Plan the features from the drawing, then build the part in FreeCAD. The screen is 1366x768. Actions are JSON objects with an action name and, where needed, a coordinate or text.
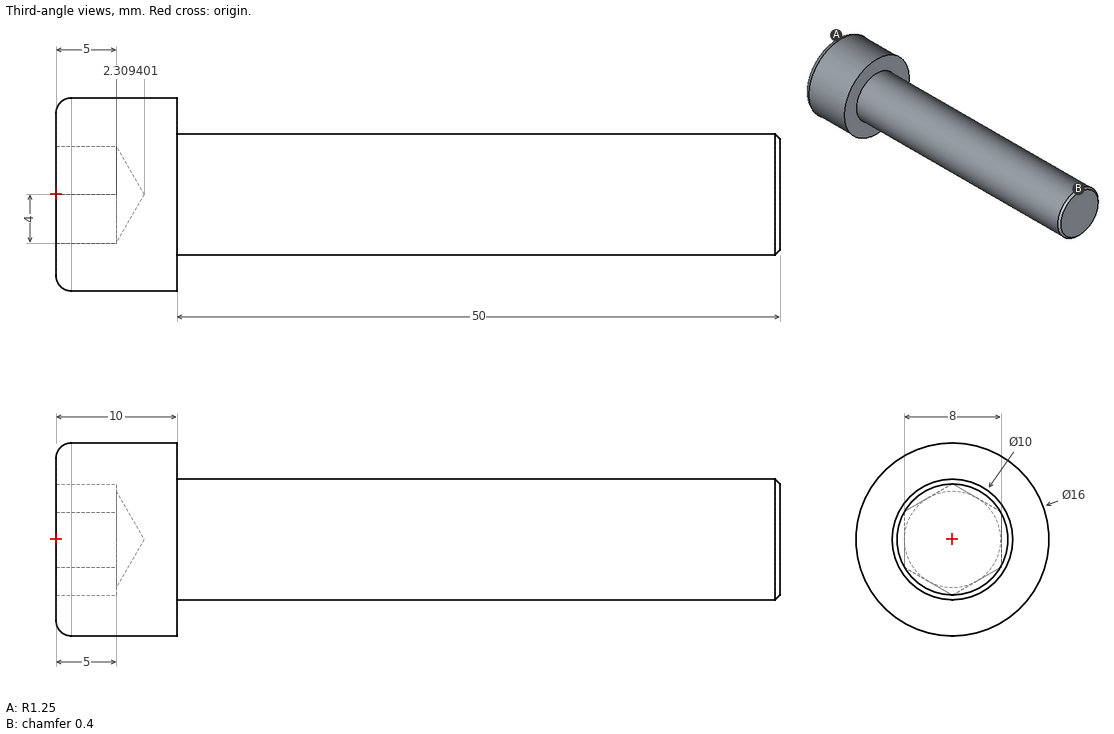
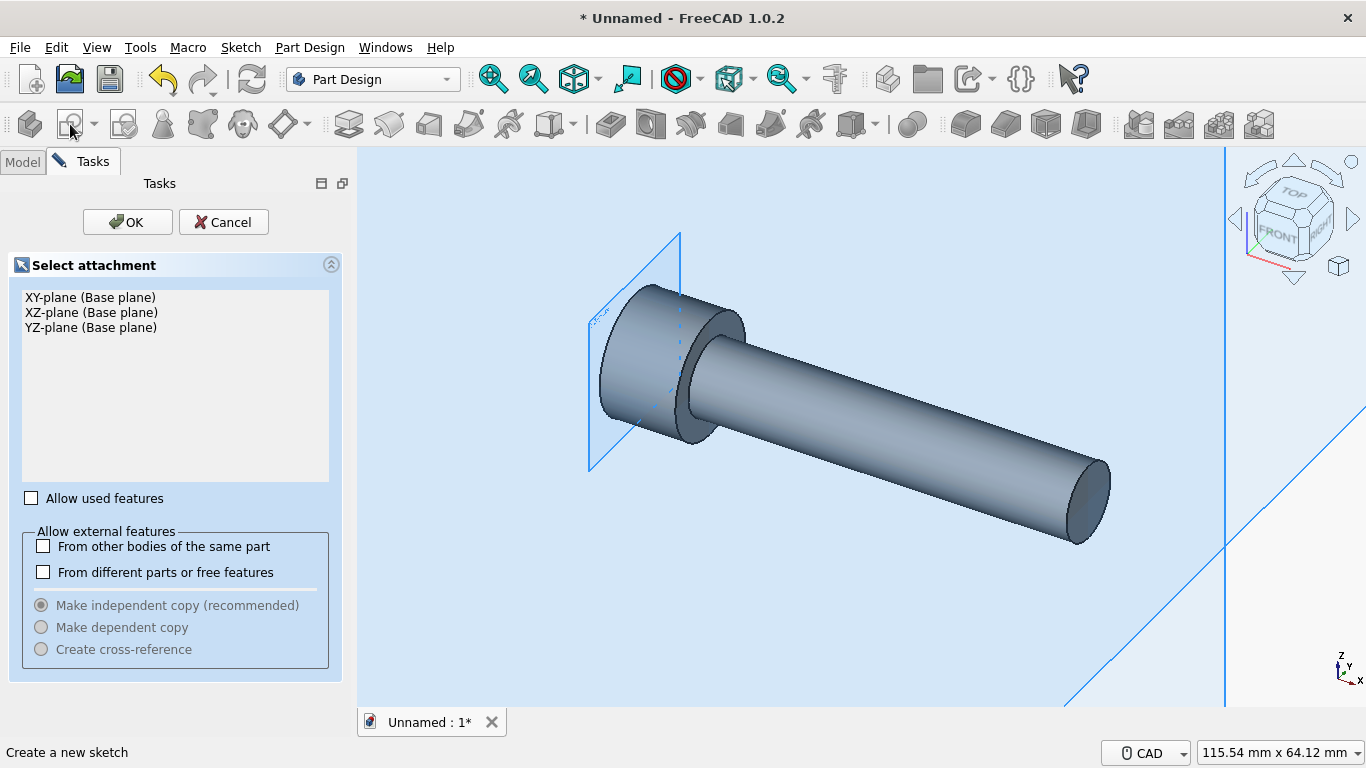
{"action": "left_click", "coordinate": [82, 328]}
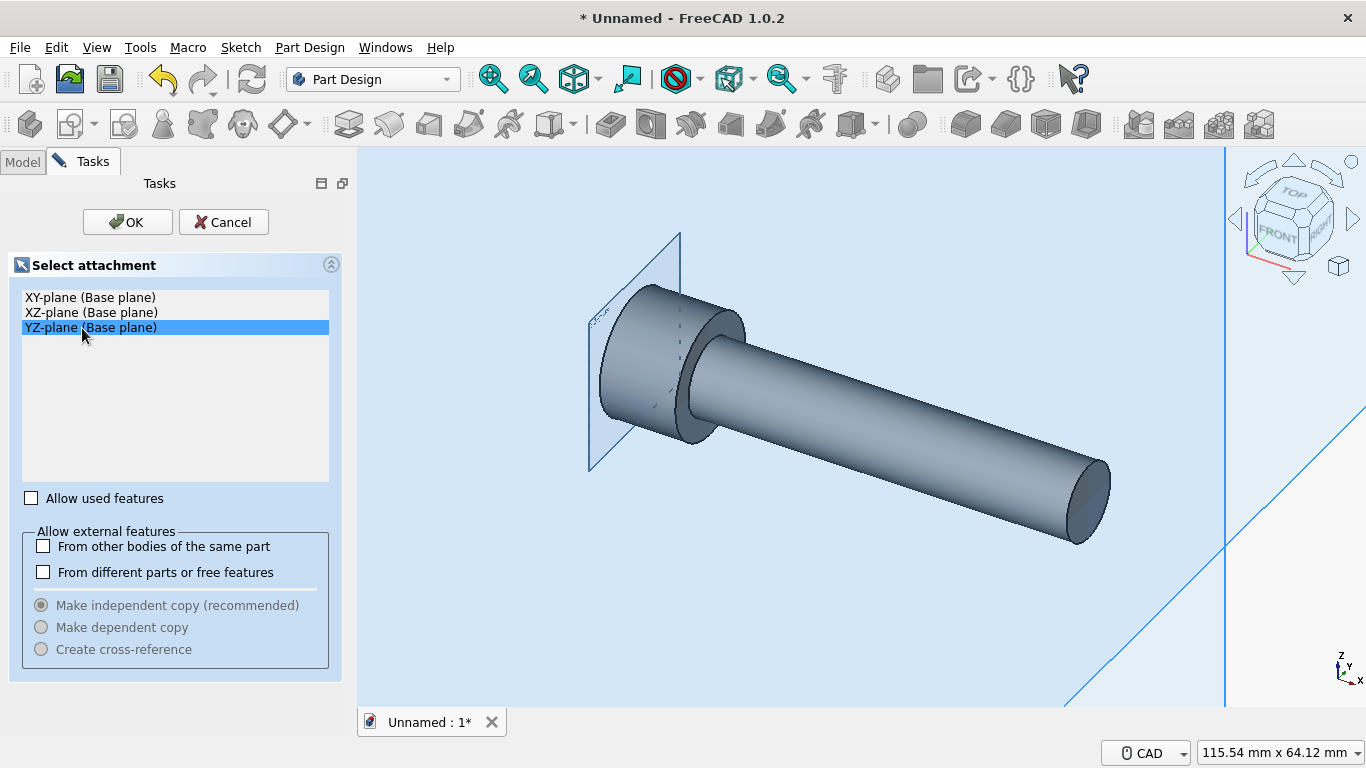
{"action": "left_click", "coordinate": [128, 222]}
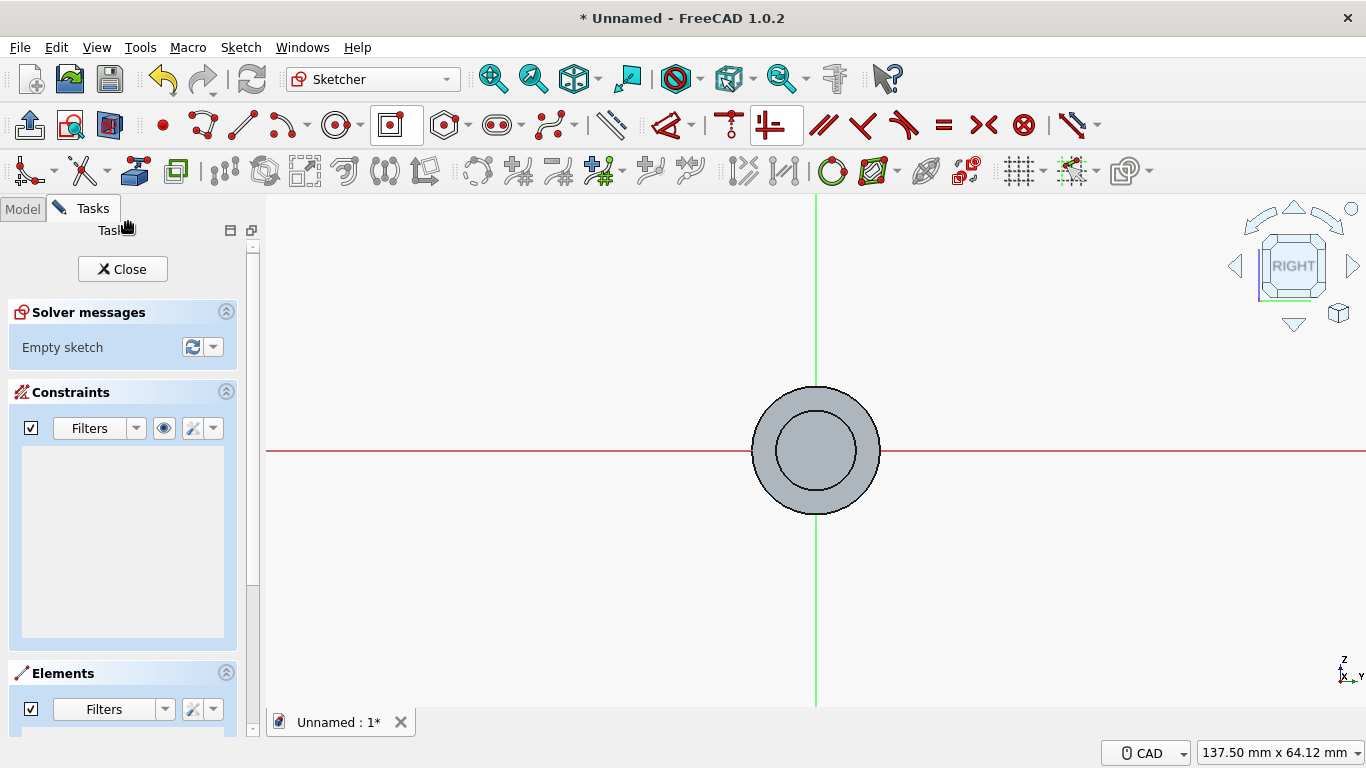
{"action": "left_click", "coordinate": [110, 126]}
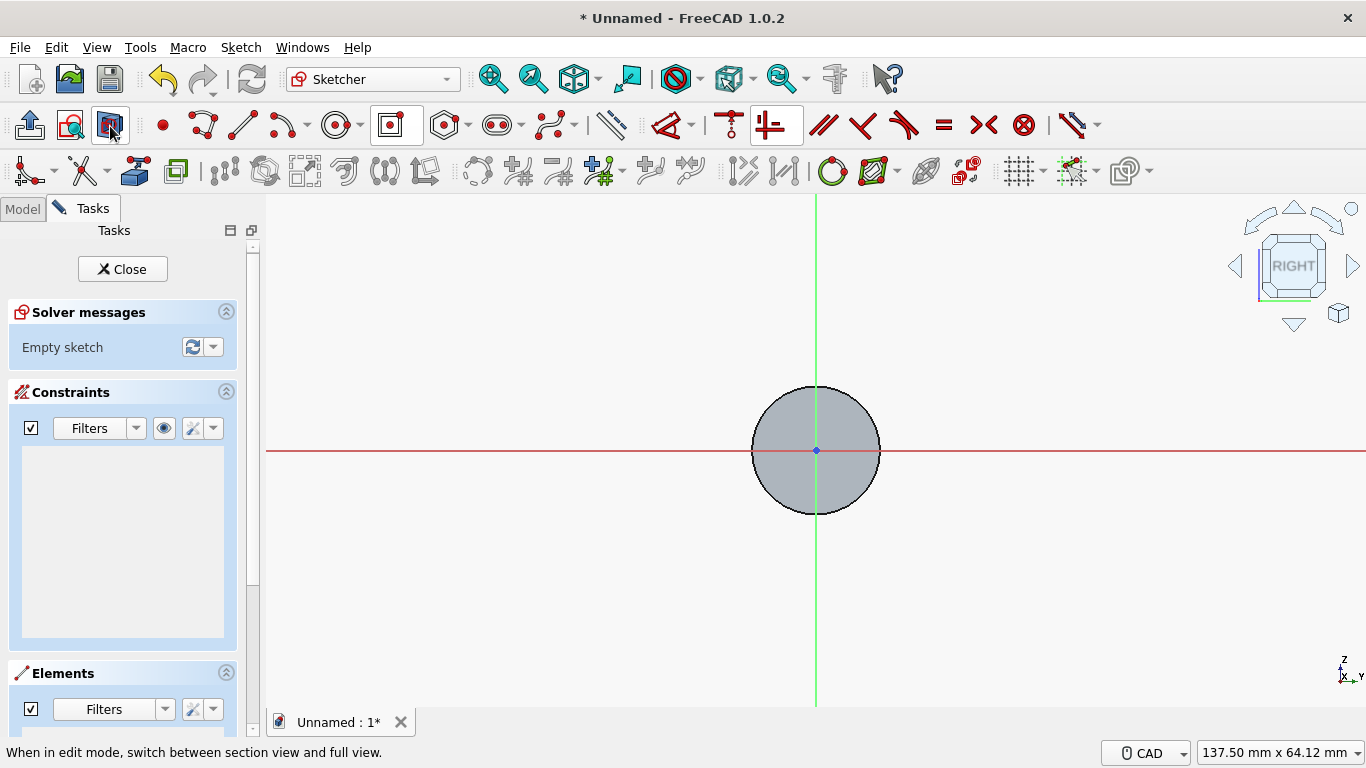
{"action": "scroll", "coordinate": [838, 450], "scroll_direction": "up", "scroll_amount": 7}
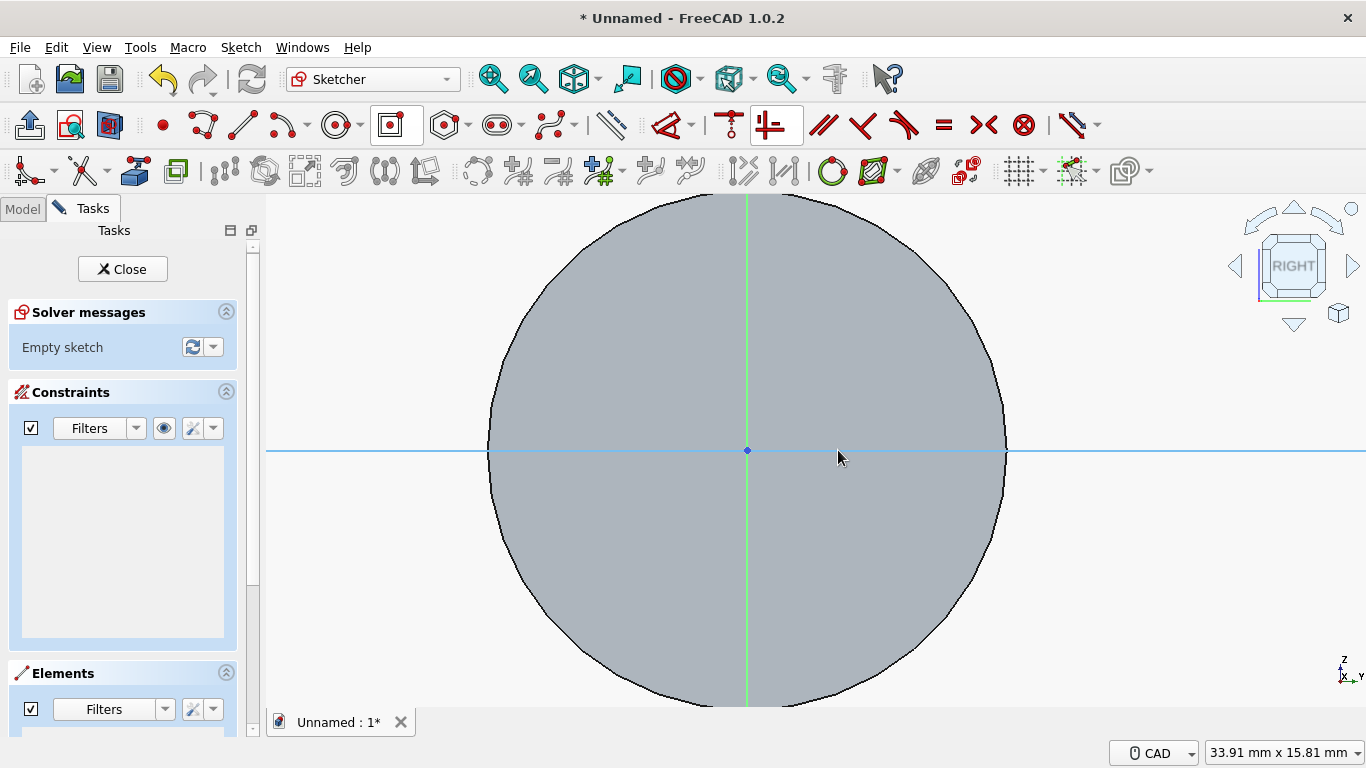
{"action": "left_click", "coordinate": [444, 126]}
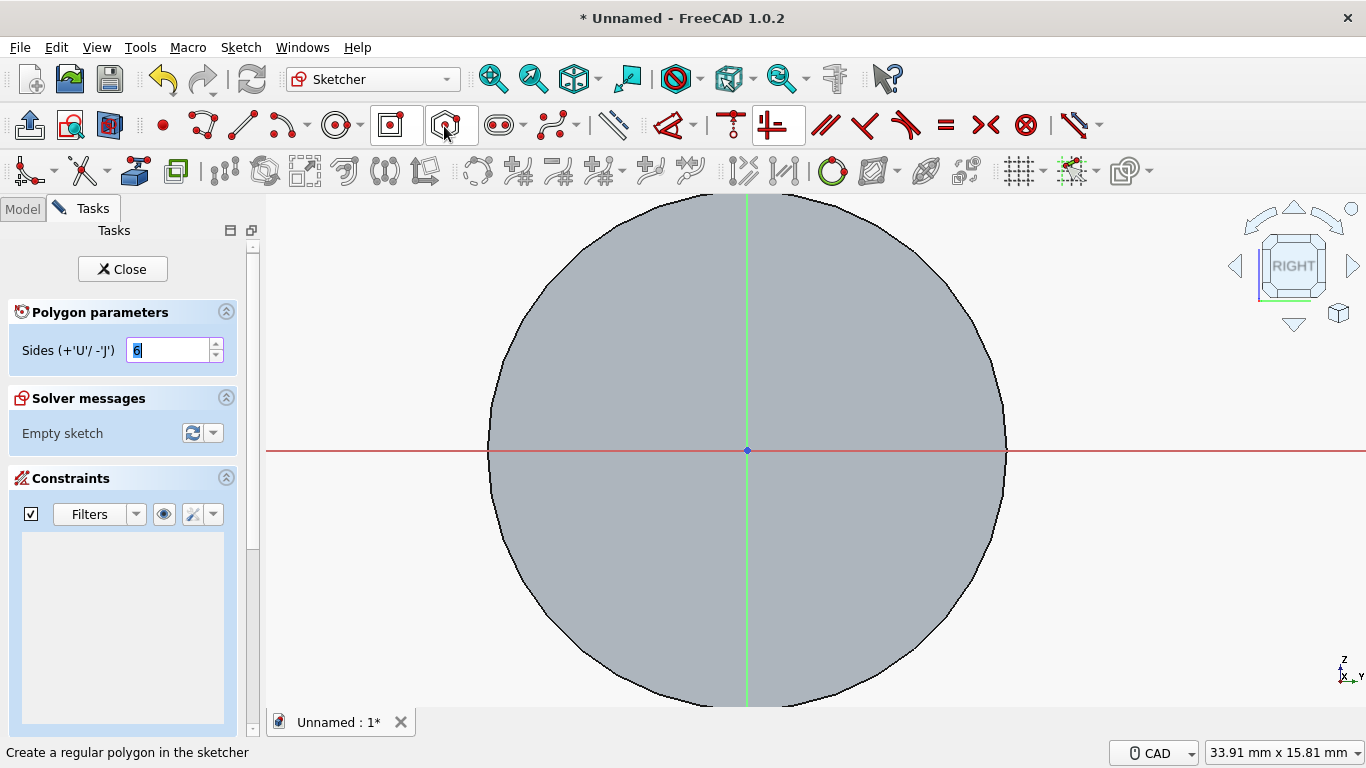
{"action": "left_click", "coordinate": [747, 450]}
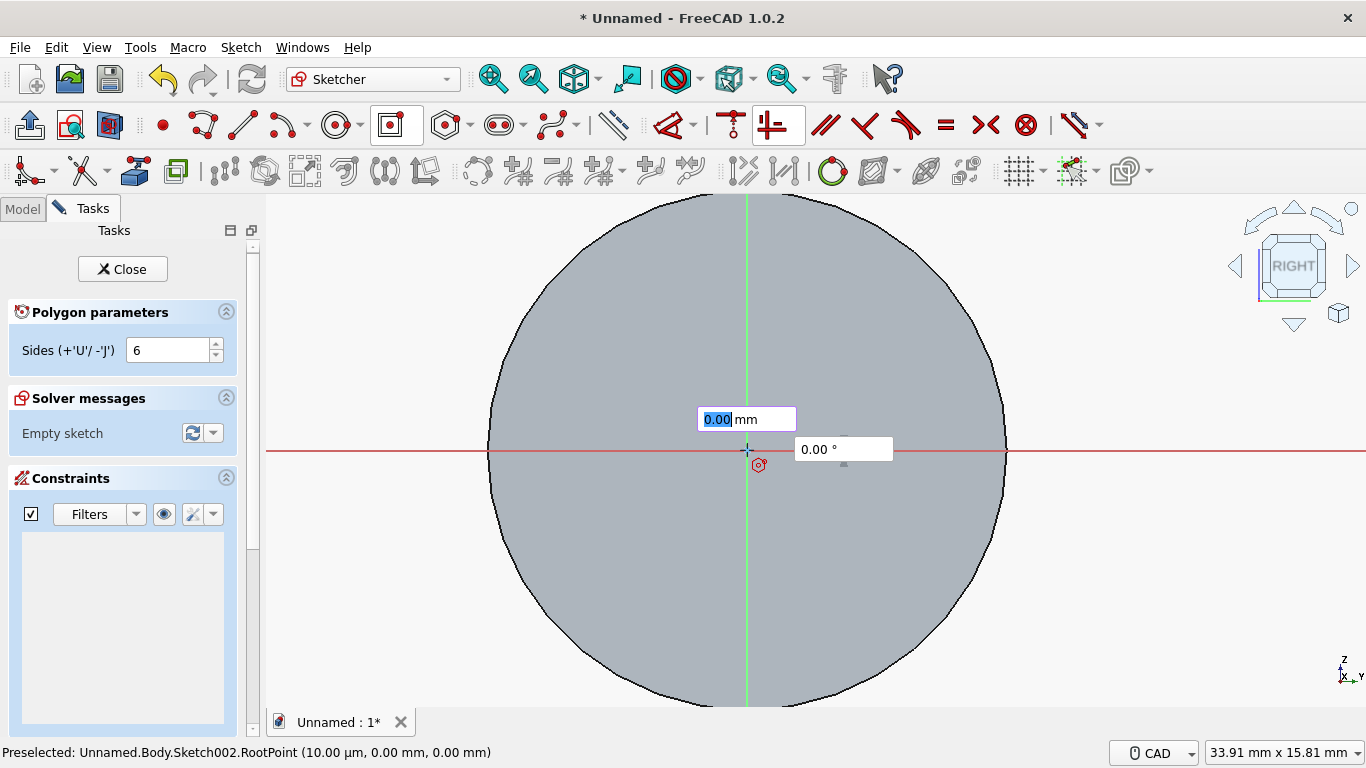
{"action": "left_click", "coordinate": [747, 600]}
{"action": "key", "text": "Escape"}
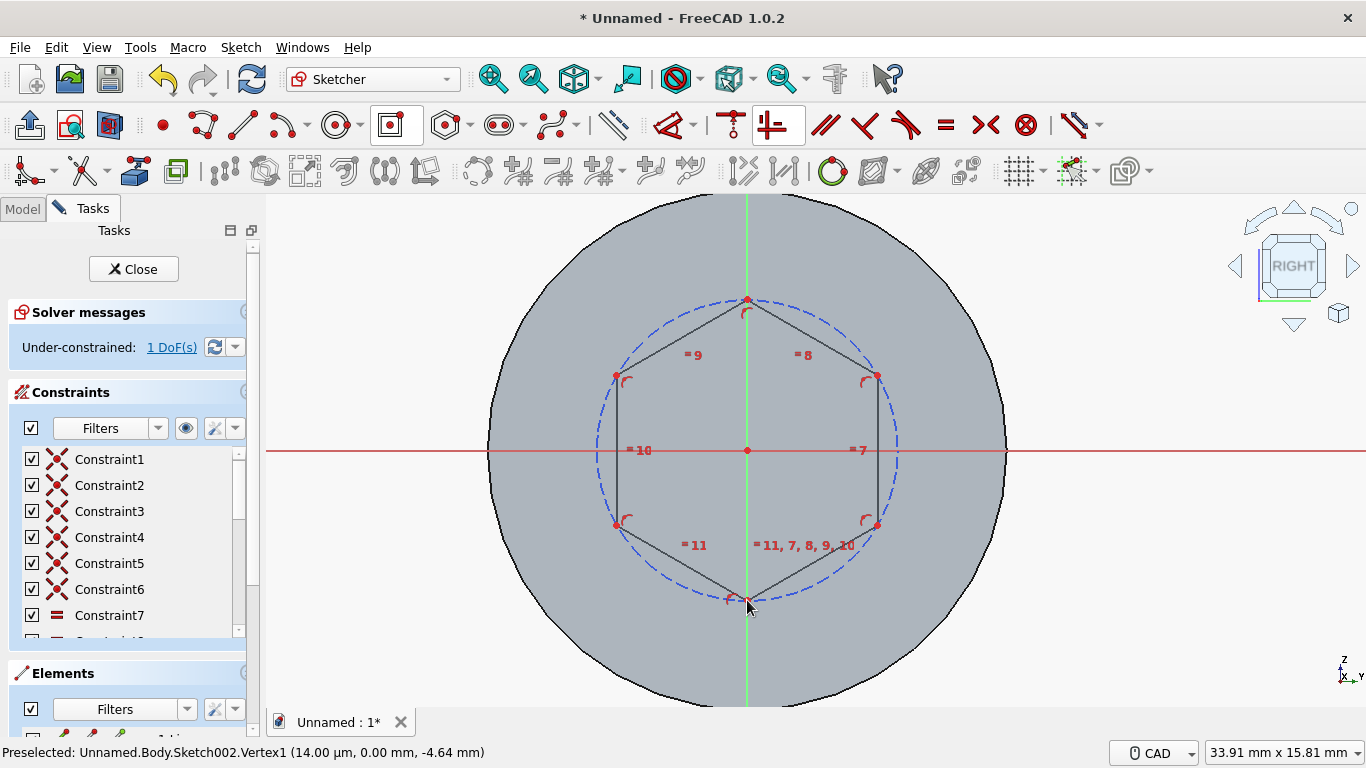
{"action": "left_click", "coordinate": [668, 126]}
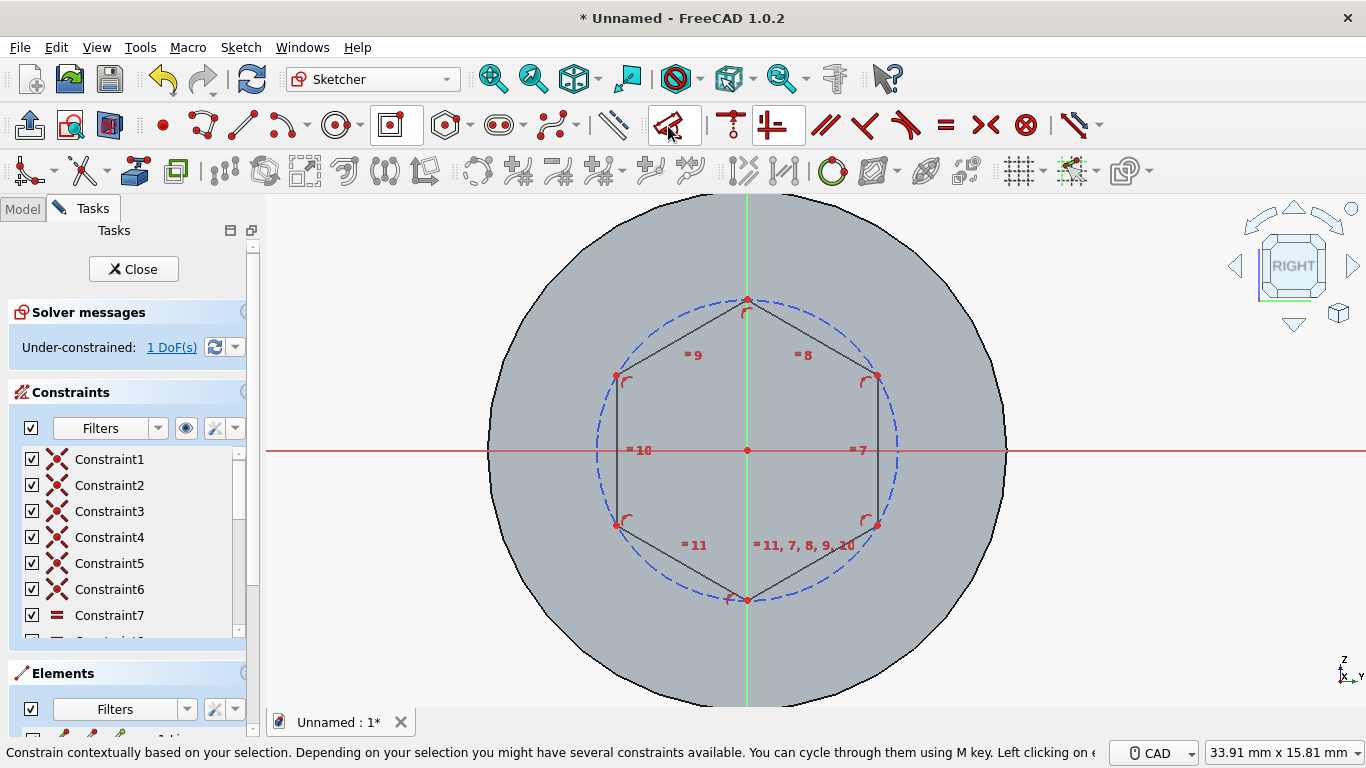
{"action": "left_click", "coordinate": [617, 375]}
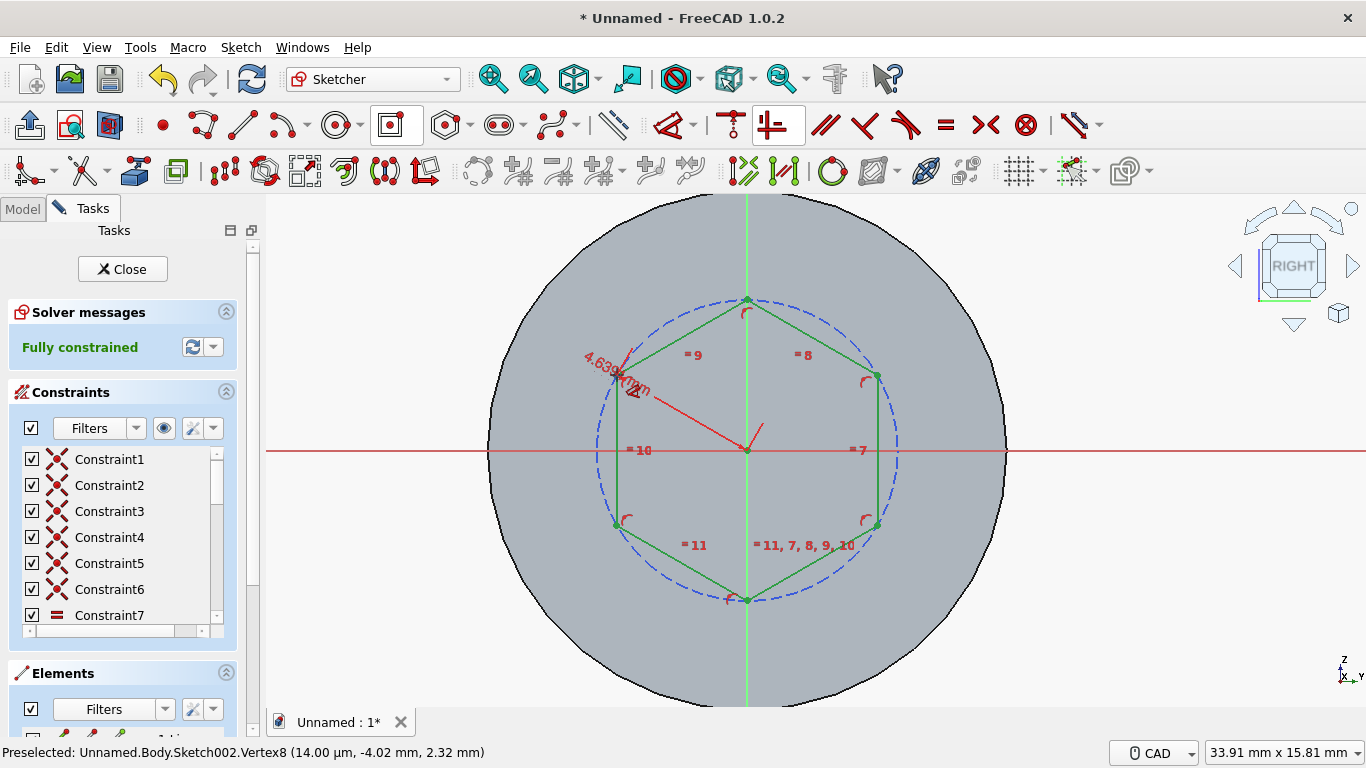
{"action": "left_click", "coordinate": [878, 526]}
{"action": "left_click", "coordinate": [687, 608]}